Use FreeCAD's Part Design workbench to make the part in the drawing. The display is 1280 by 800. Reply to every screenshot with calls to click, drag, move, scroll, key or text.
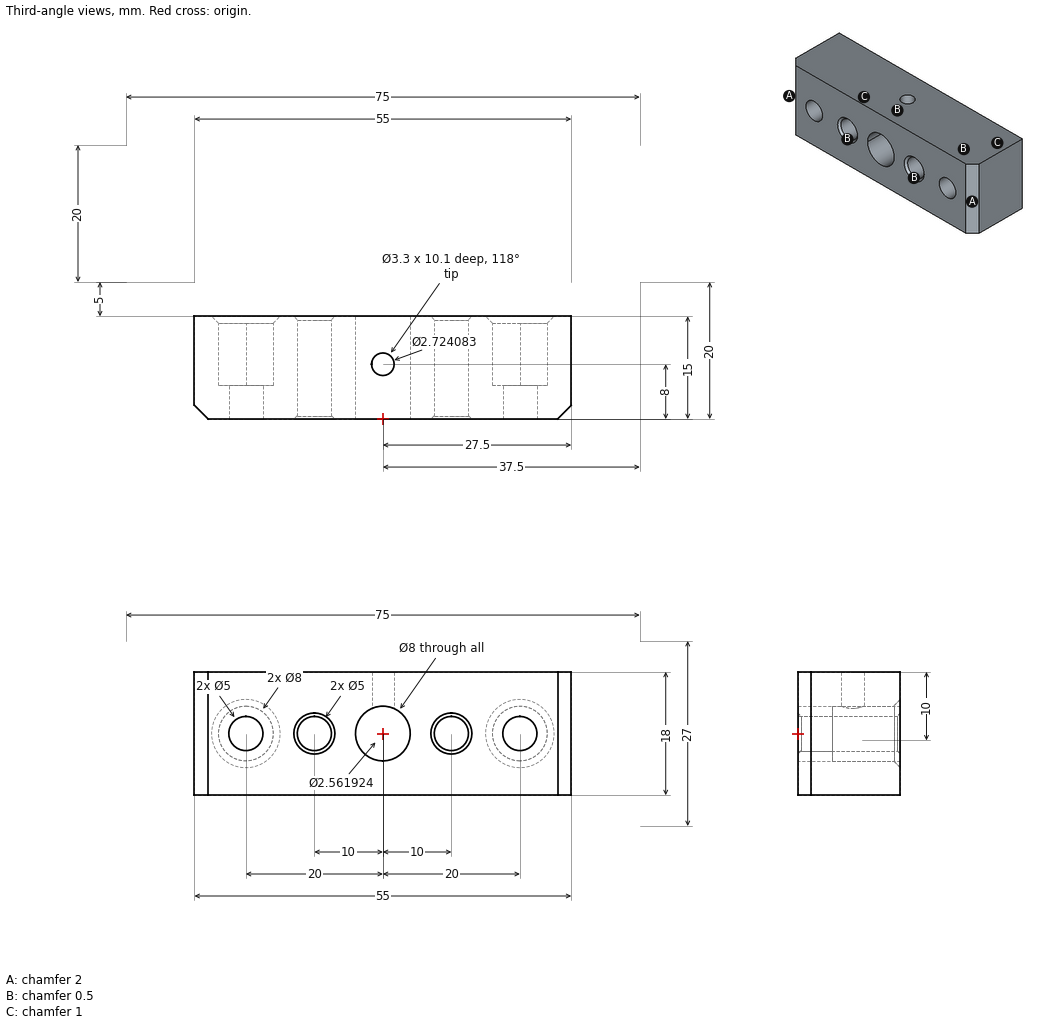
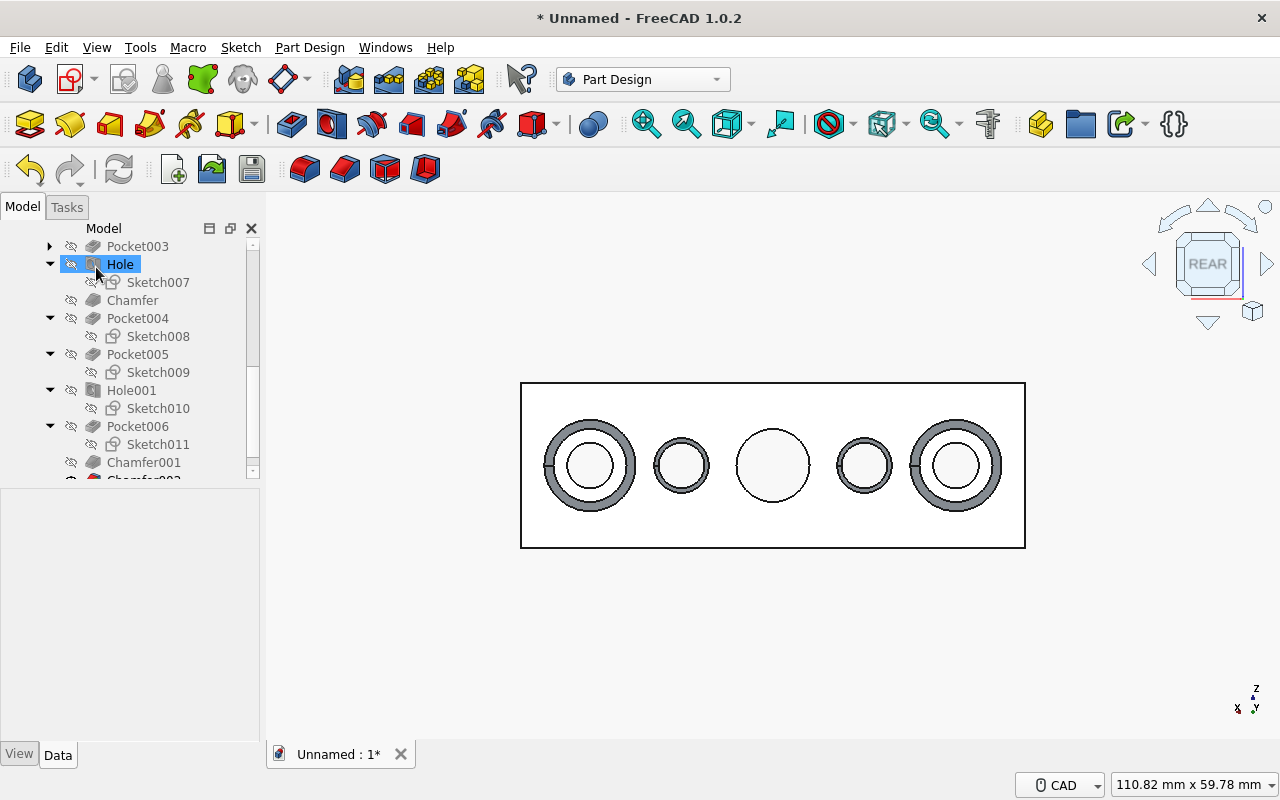
key(0)